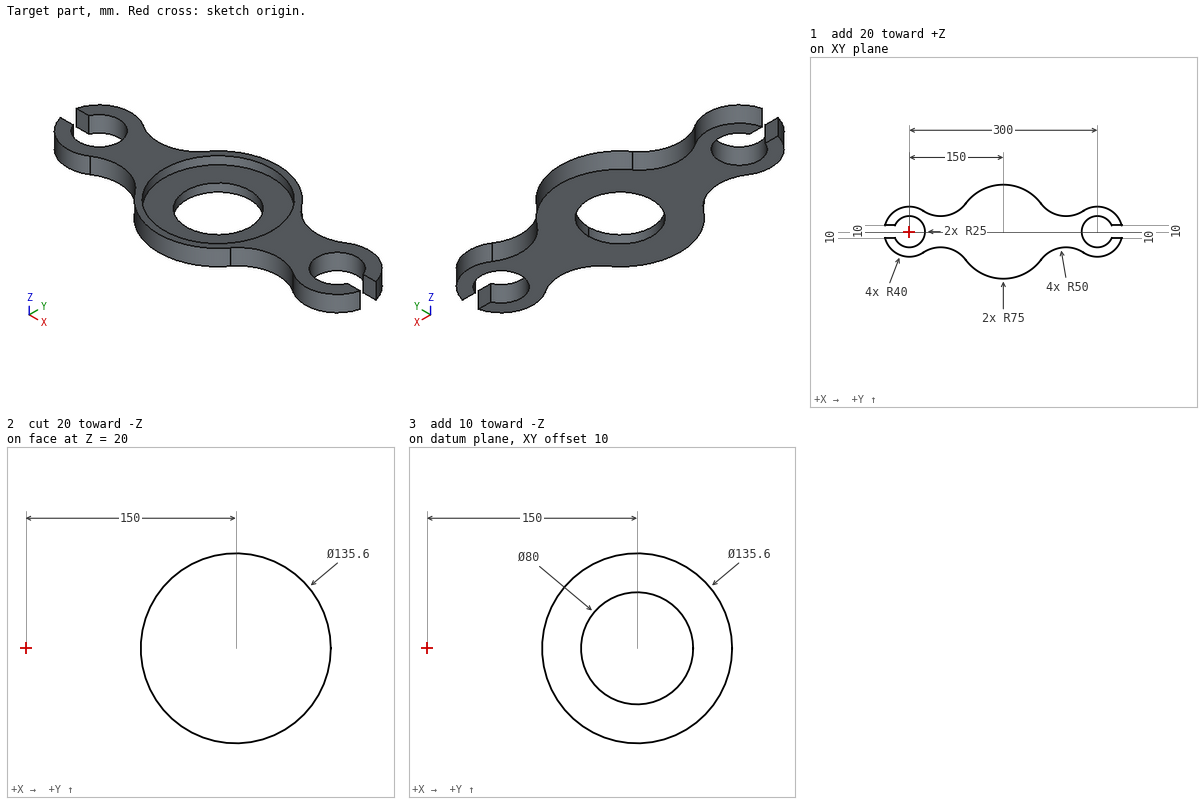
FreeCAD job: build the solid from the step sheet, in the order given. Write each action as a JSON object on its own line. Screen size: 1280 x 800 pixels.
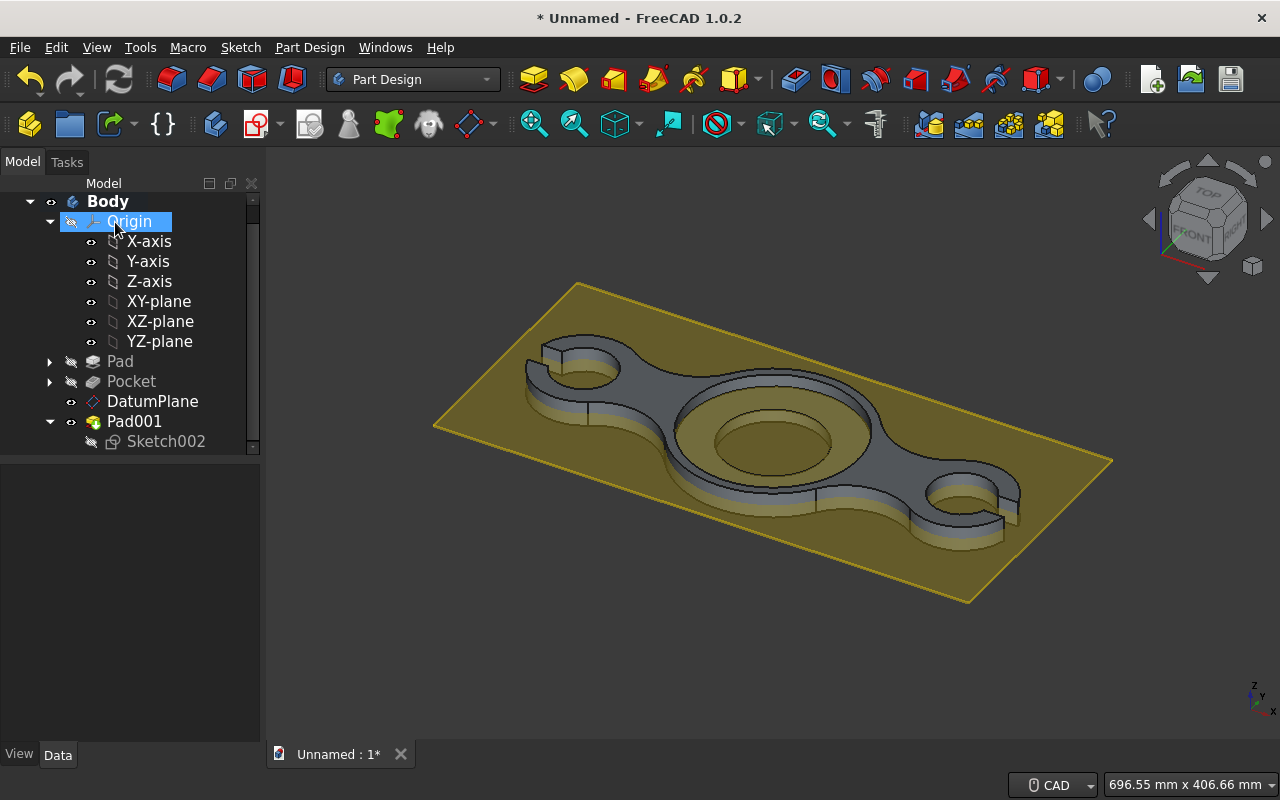
{"action": "left_click", "coordinate": [116, 402]}
{"action": "key", "text": "space"}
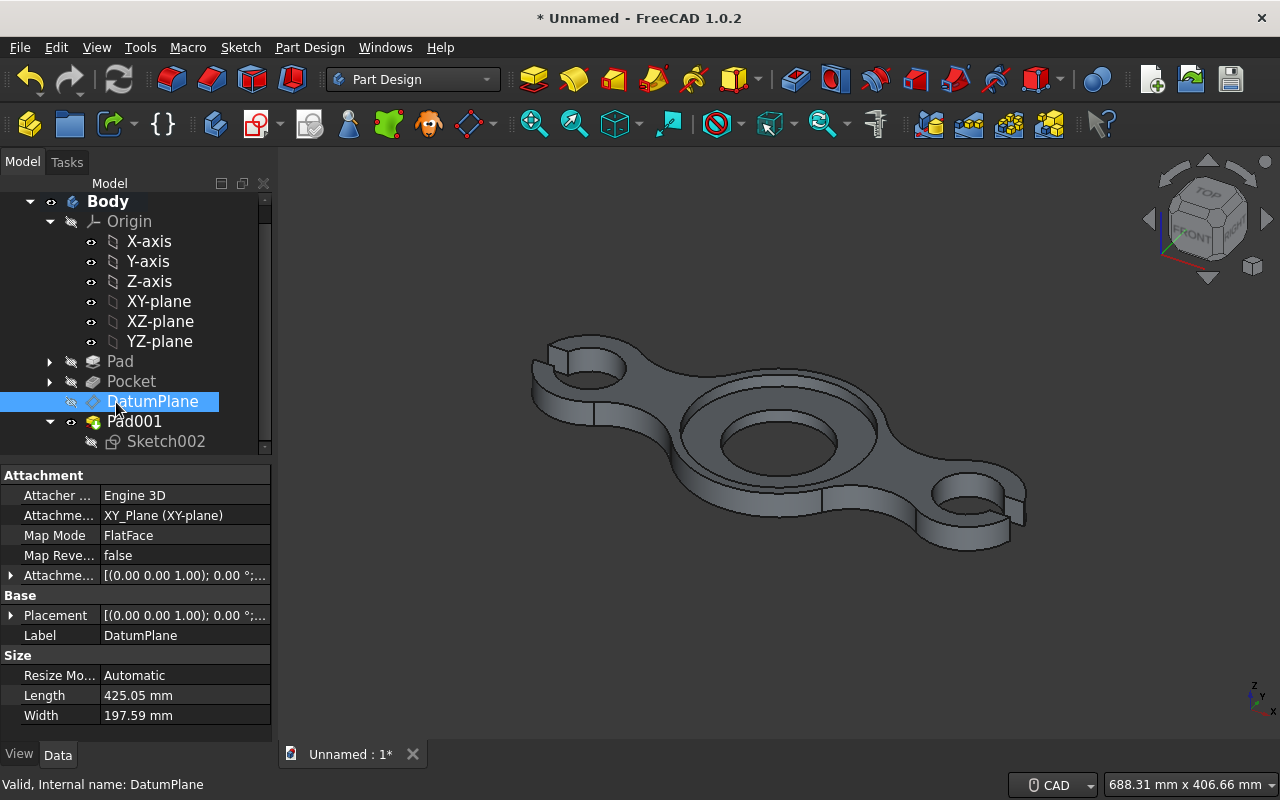
{"action": "key", "text": "0"}